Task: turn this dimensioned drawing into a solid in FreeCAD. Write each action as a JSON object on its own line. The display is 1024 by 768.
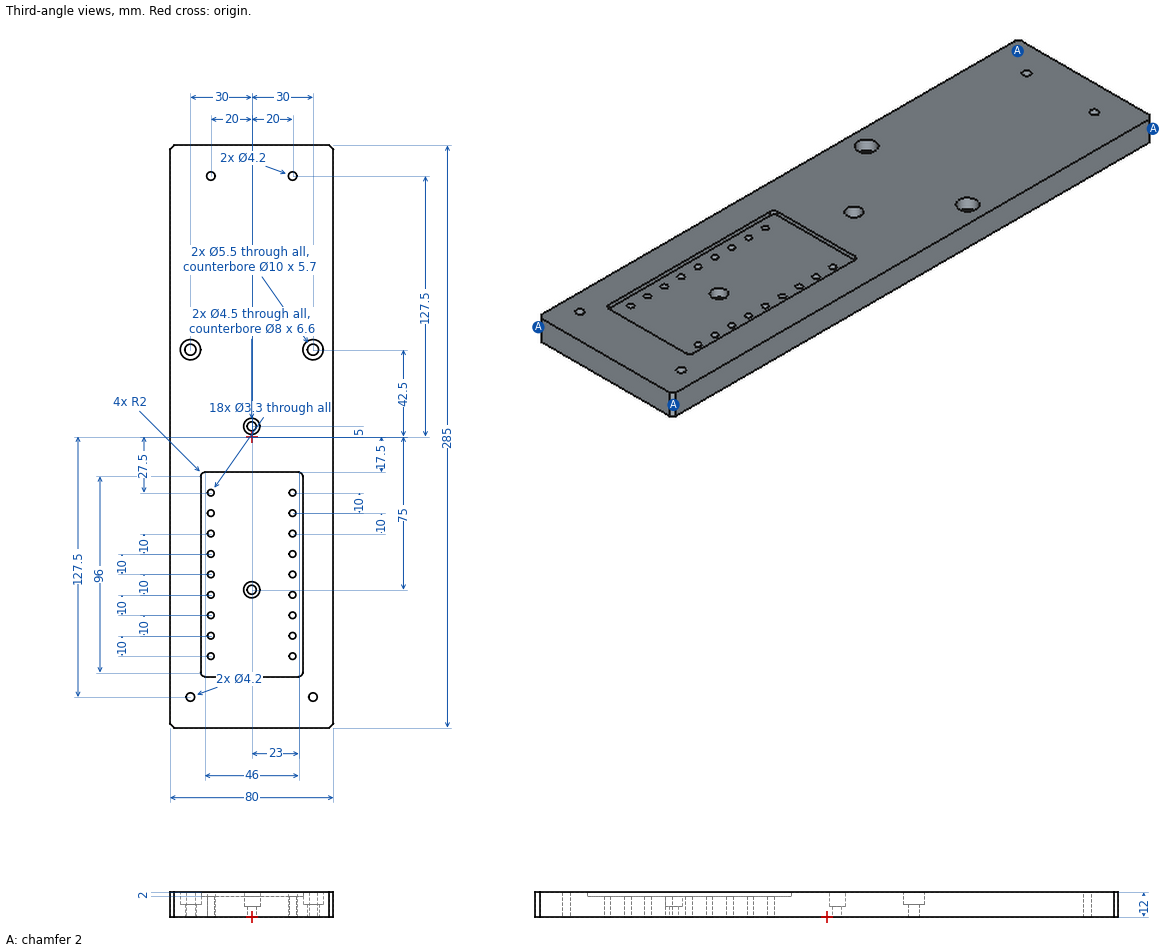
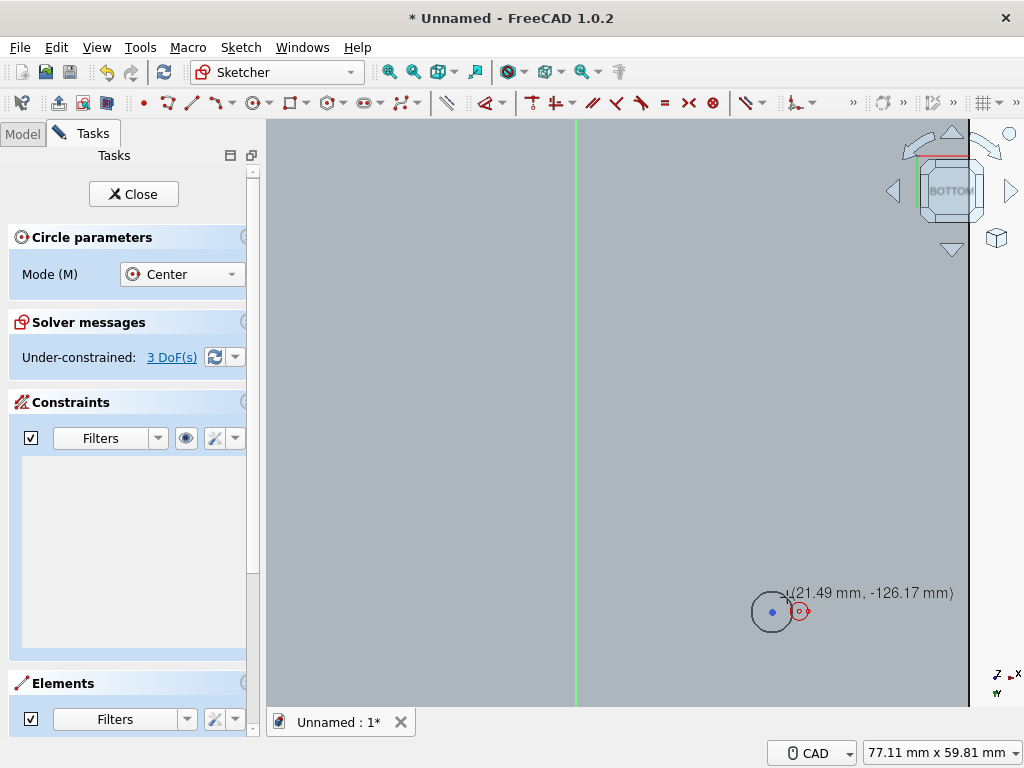
{"action": "left_click", "coordinate": [379, 611]}
{"action": "left_click", "coordinate": [394, 597]}
{"action": "key", "text": "Escape"}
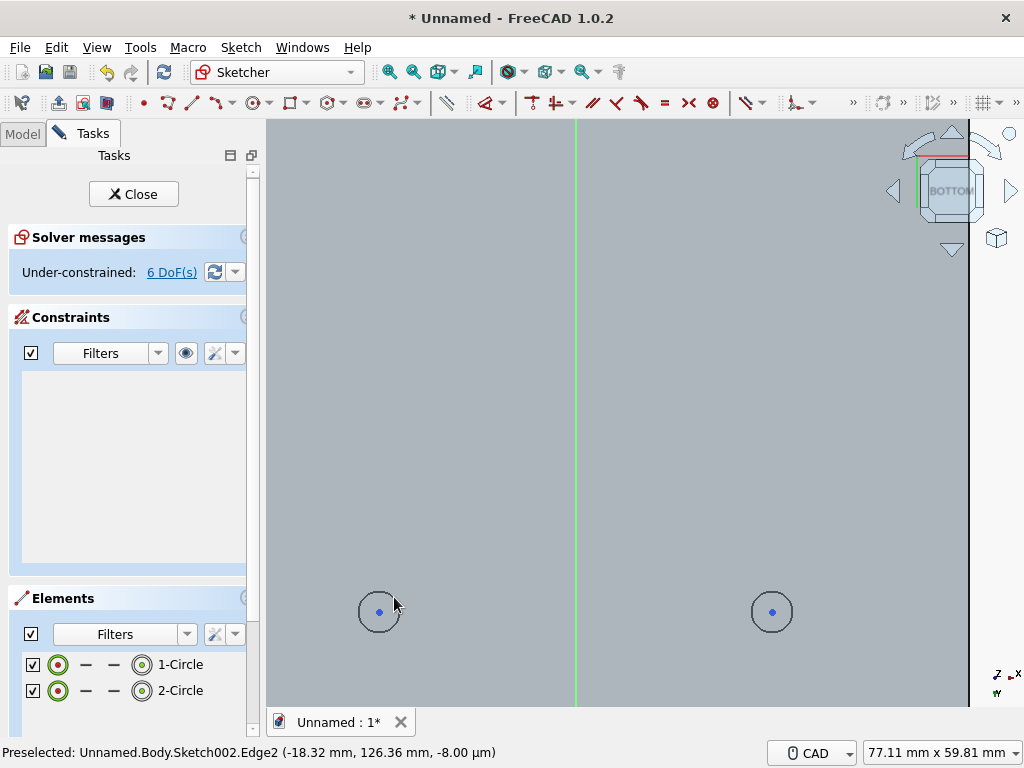
{"action": "left_click", "coordinate": [786, 597]}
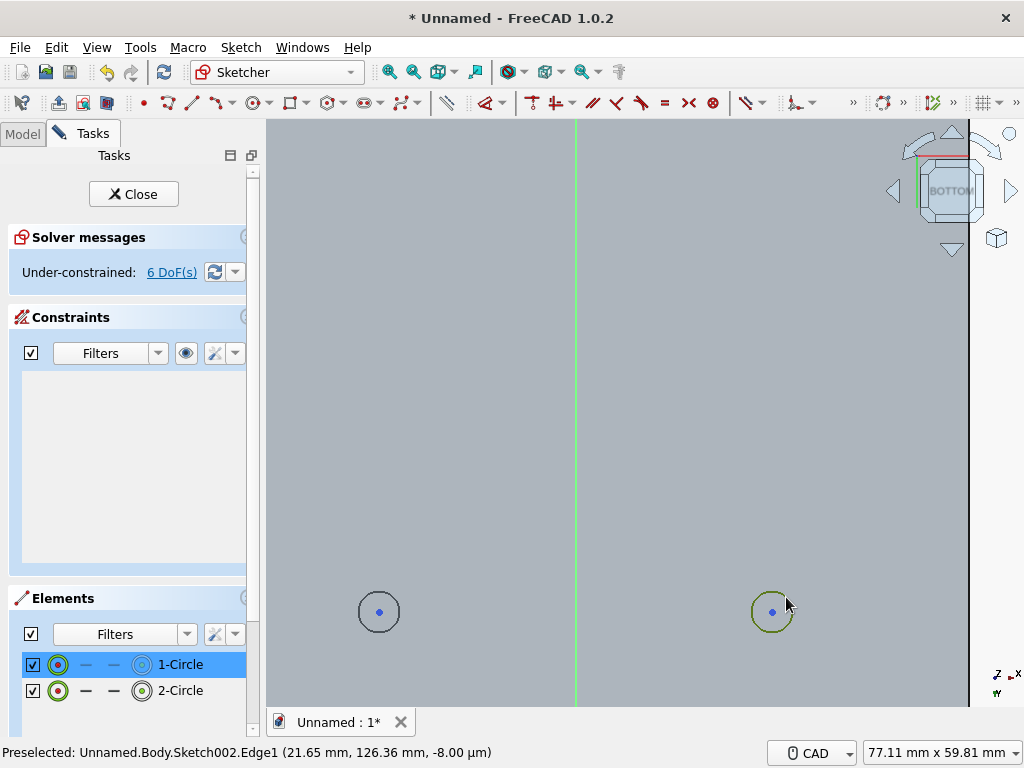
{"action": "left_click", "coordinate": [393, 597]}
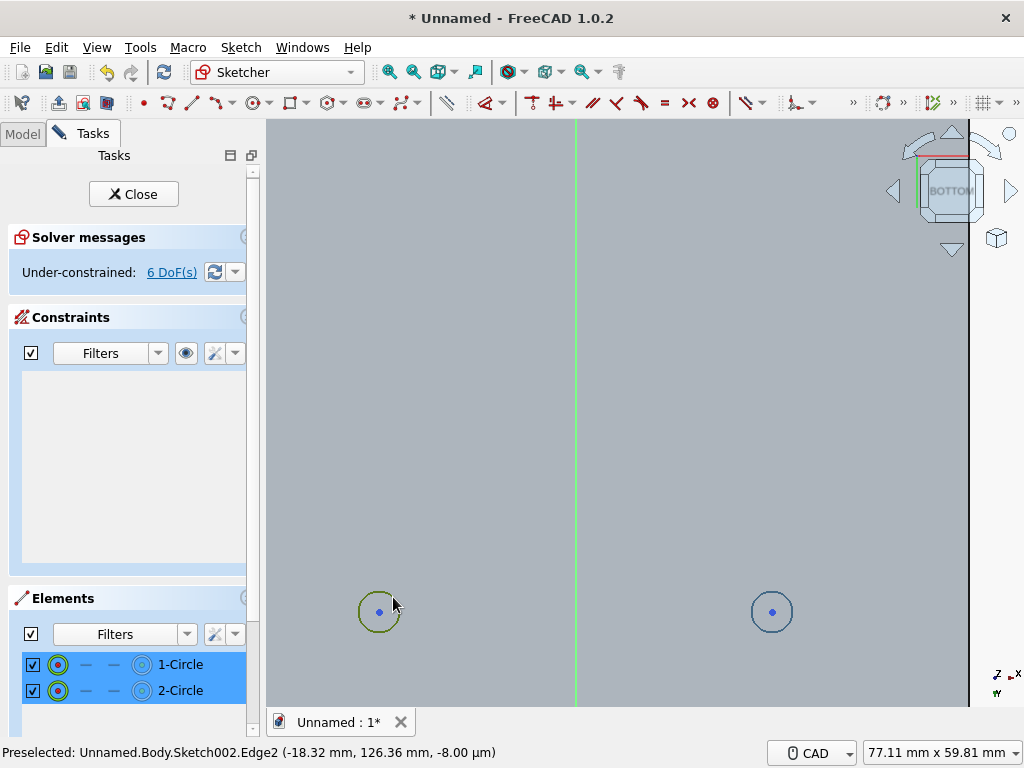
{"action": "left_click", "coordinate": [666, 104]}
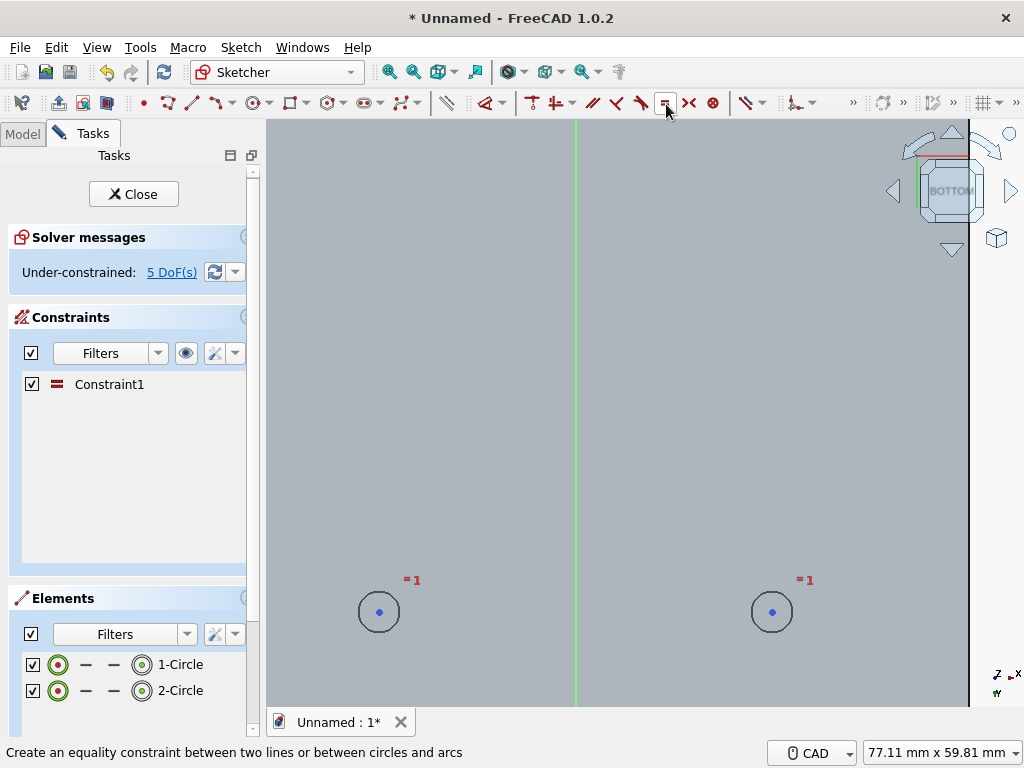
{"action": "left_click", "coordinate": [772, 612]}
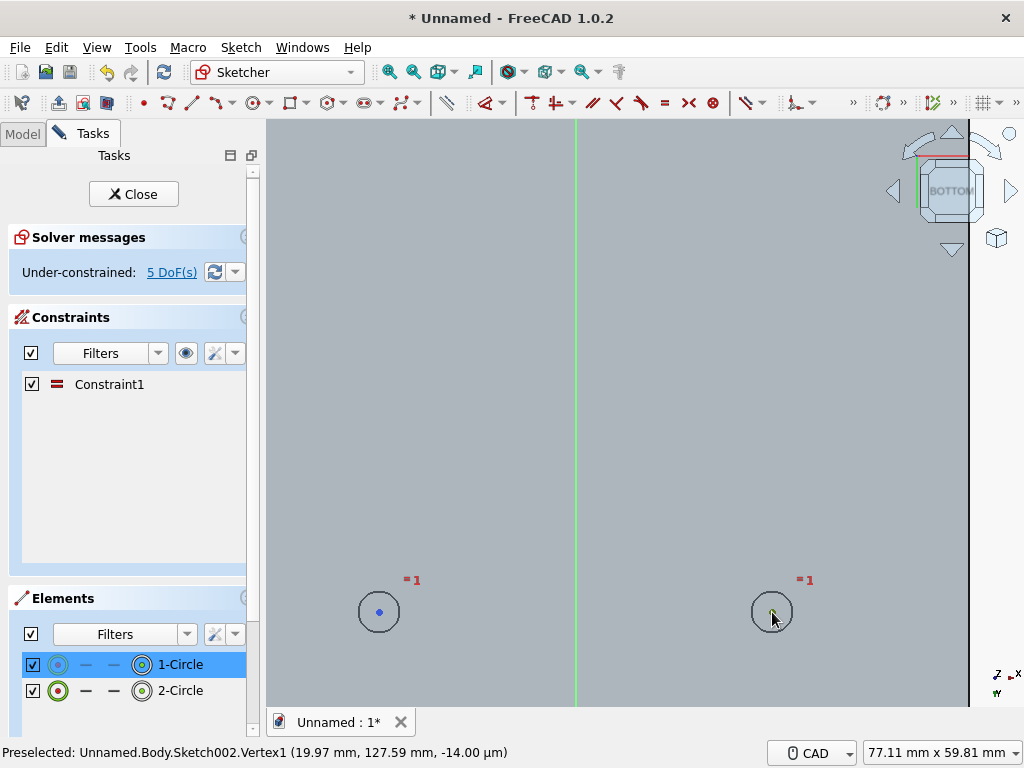
{"action": "left_click", "coordinate": [379, 612]}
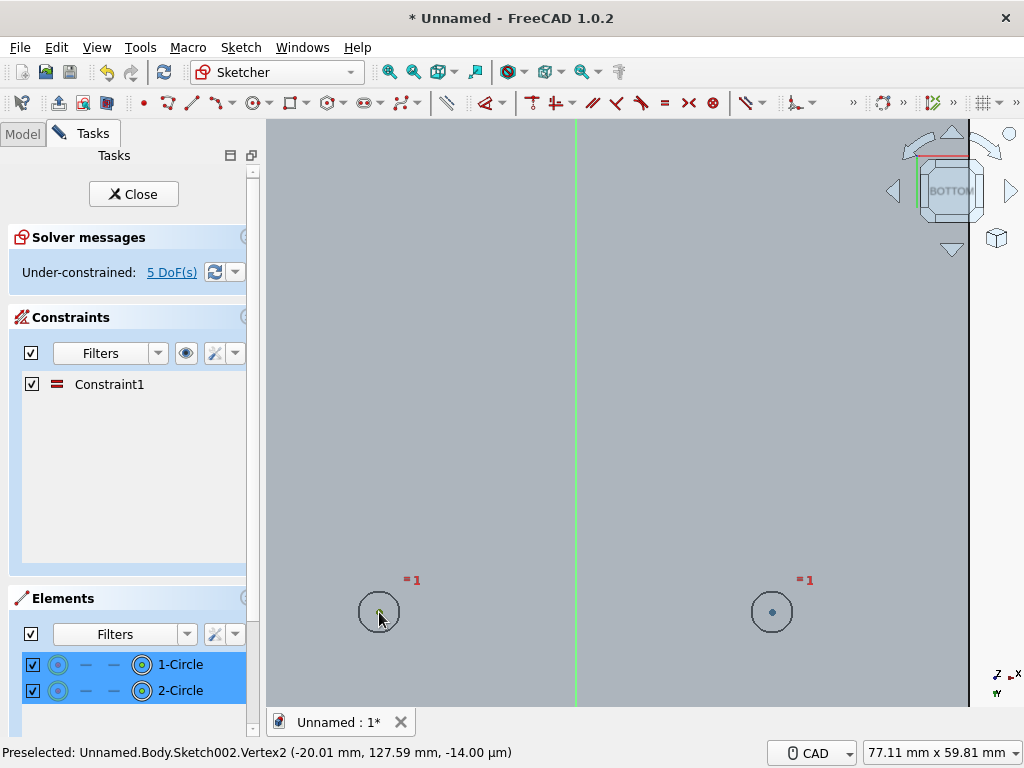
{"action": "key", "text": "h"}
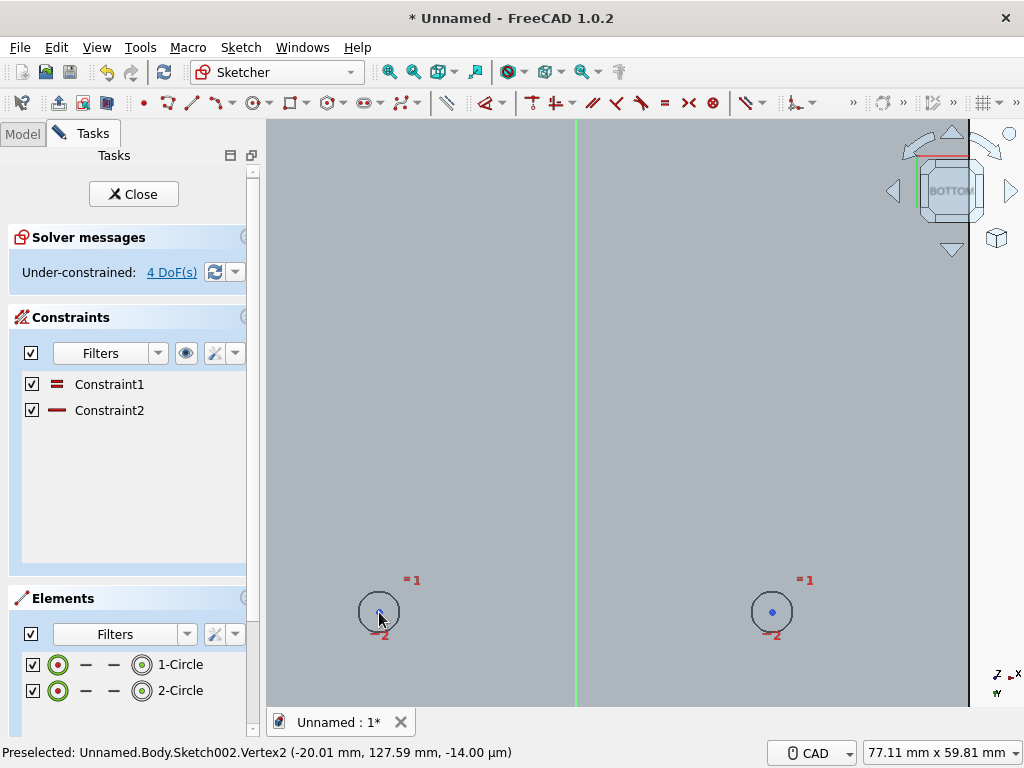
{"action": "key", "text": "d"}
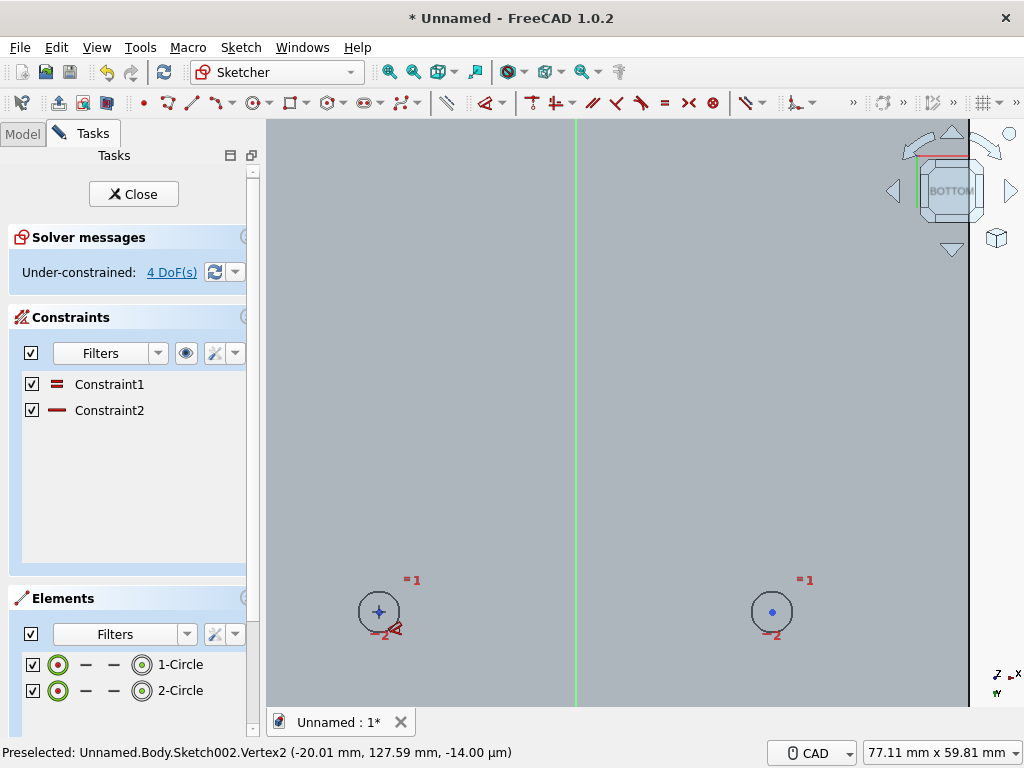
{"action": "left_click", "coordinate": [786, 597]}
{"action": "left_click", "coordinate": [808, 574]}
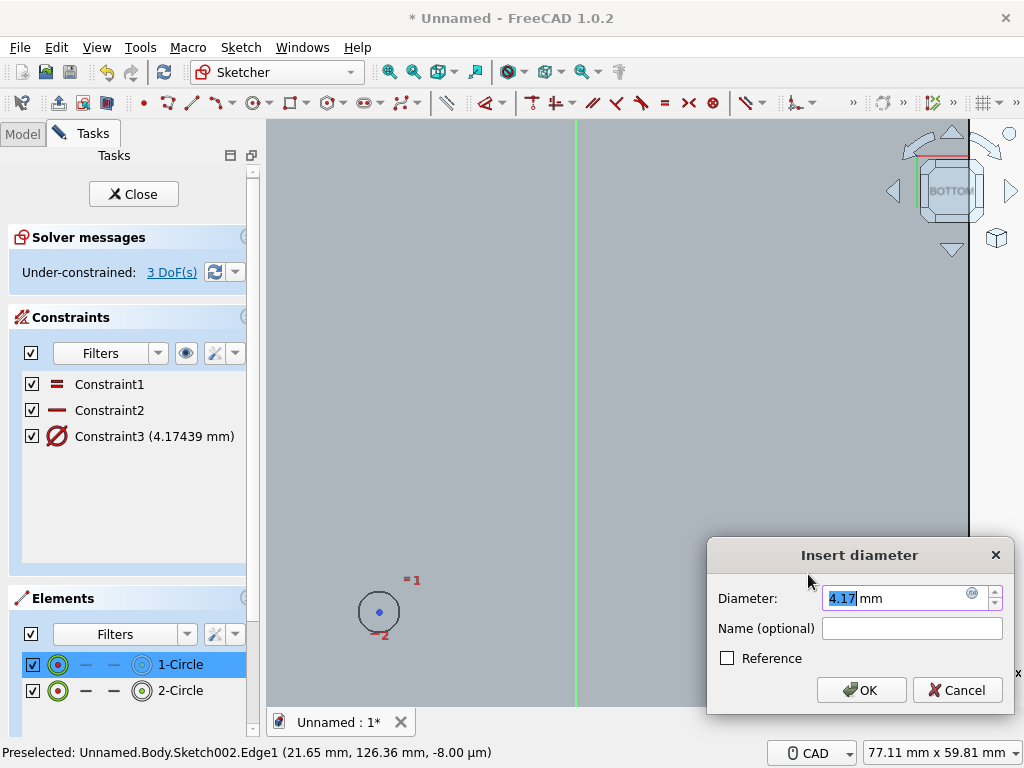
{"action": "type", "text": "4.2"}
{"action": "key", "text": "Return"}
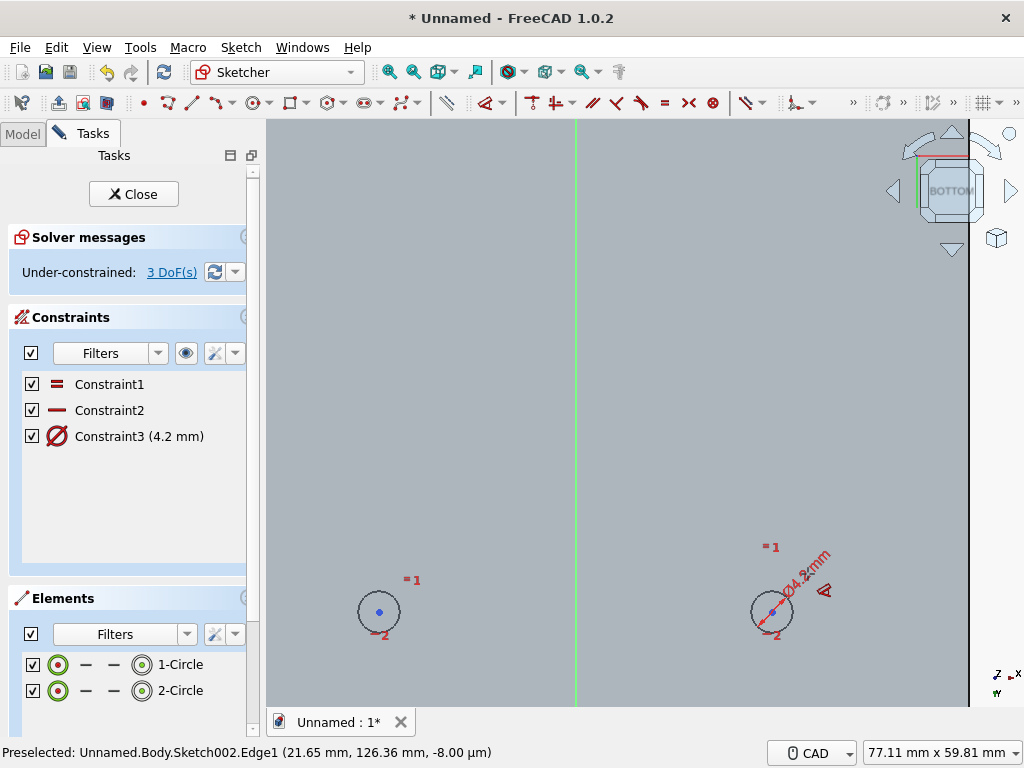
{"action": "left_click", "coordinate": [772, 612]}
{"action": "left_click", "coordinate": [674, 646]}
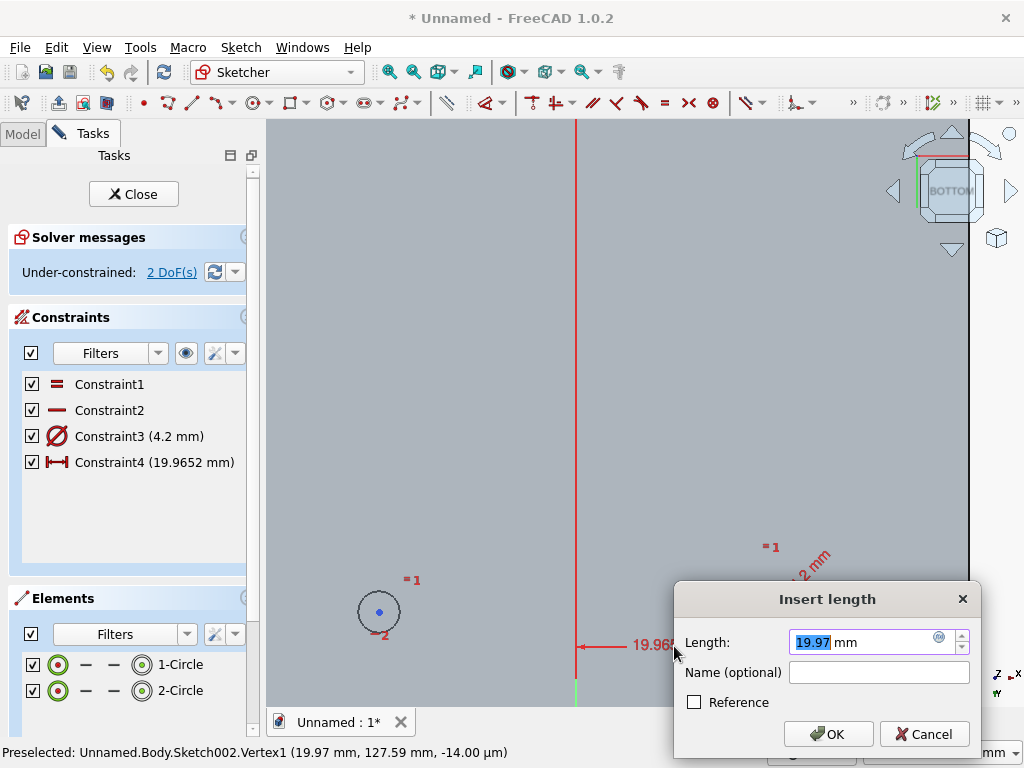
{"action": "type", "text": "20"}
{"action": "key", "text": "Return"}